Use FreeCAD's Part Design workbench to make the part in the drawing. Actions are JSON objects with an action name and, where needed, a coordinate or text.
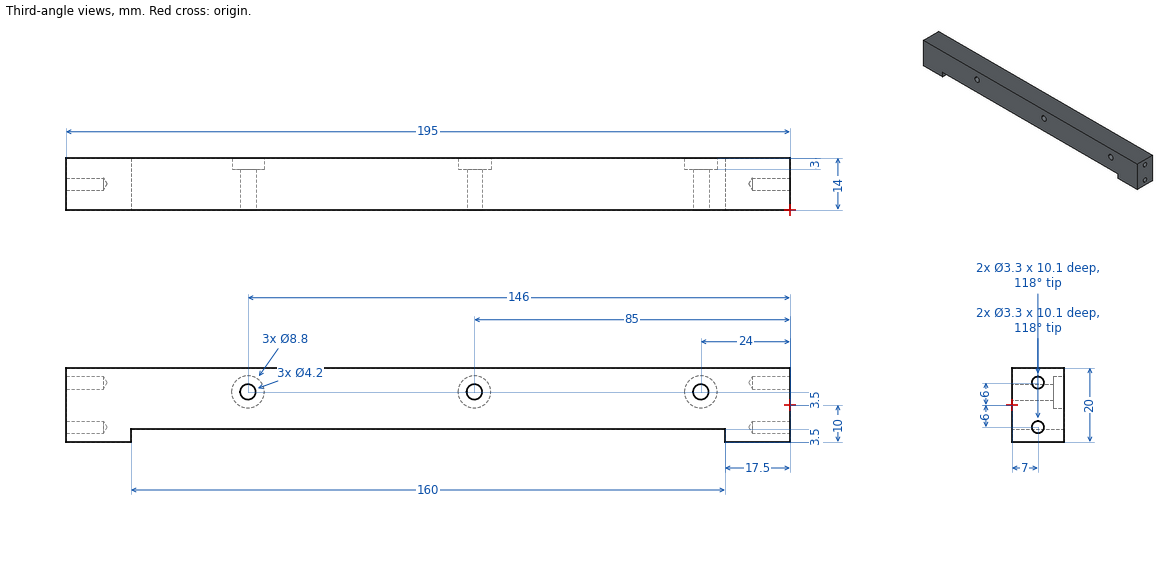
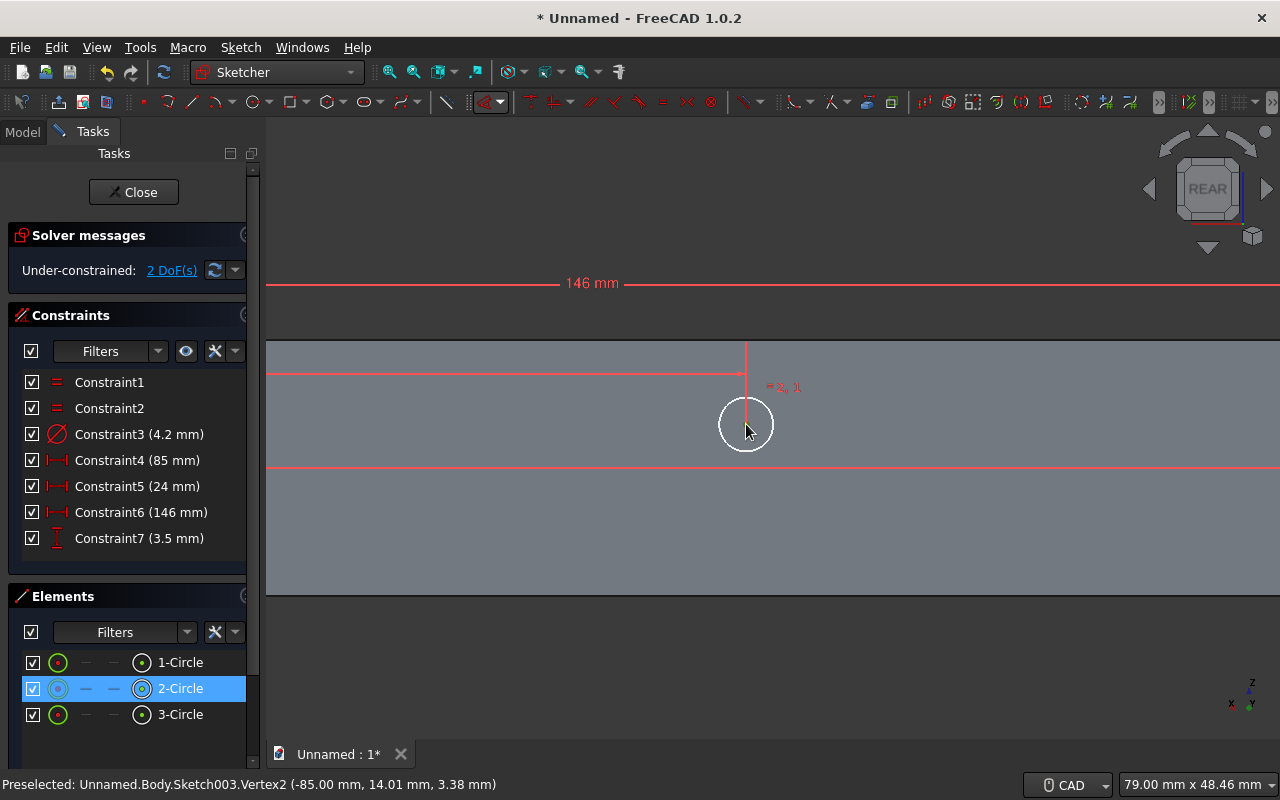
{"action": "left_click", "coordinate": [502, 102]}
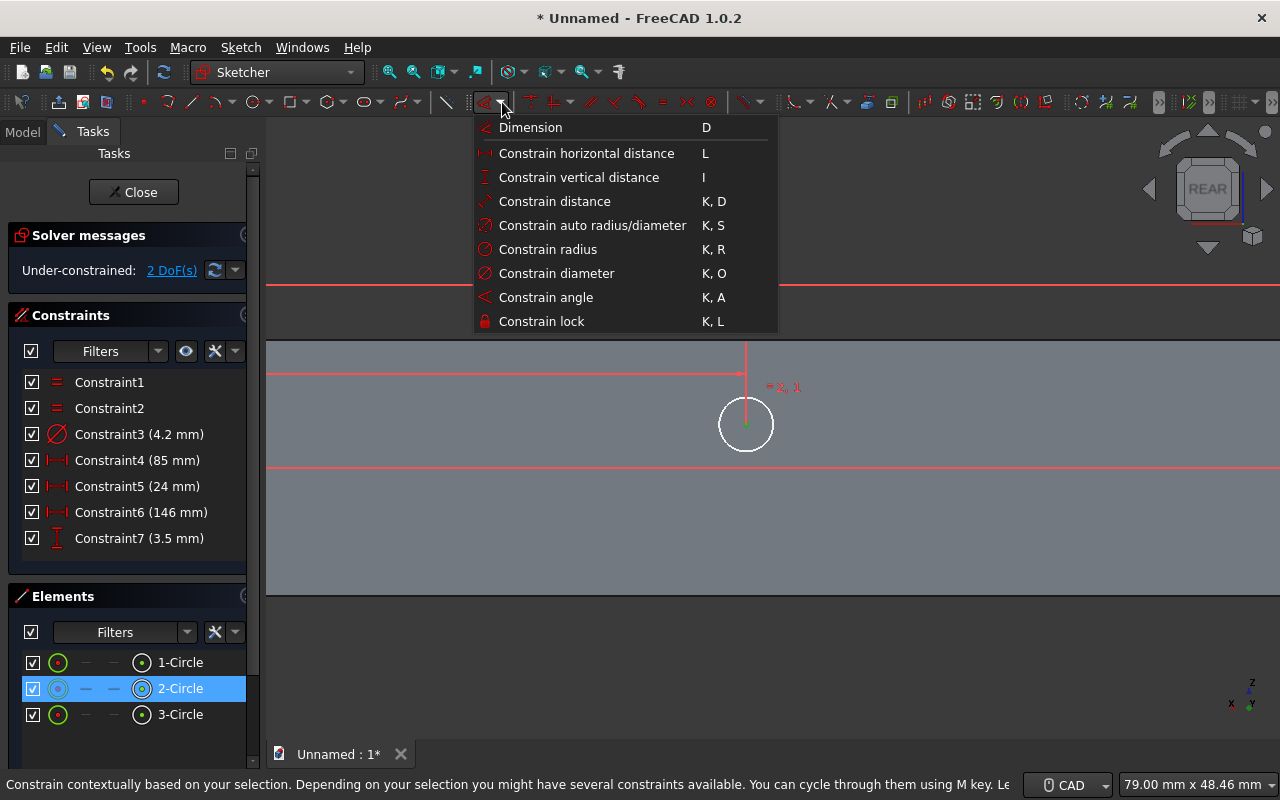
{"action": "left_click", "coordinate": [626, 177]}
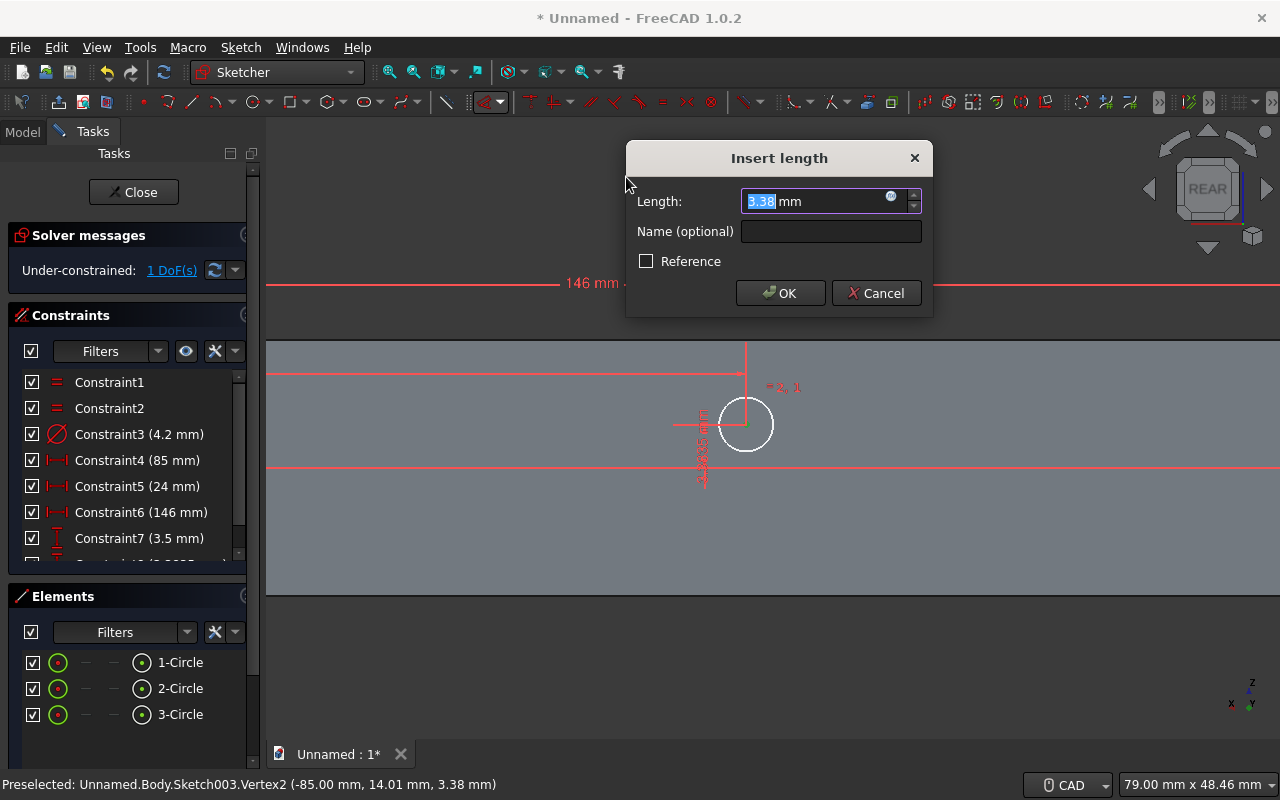
{"action": "type", "text": "3.5"}
{"action": "key", "text": "Return"}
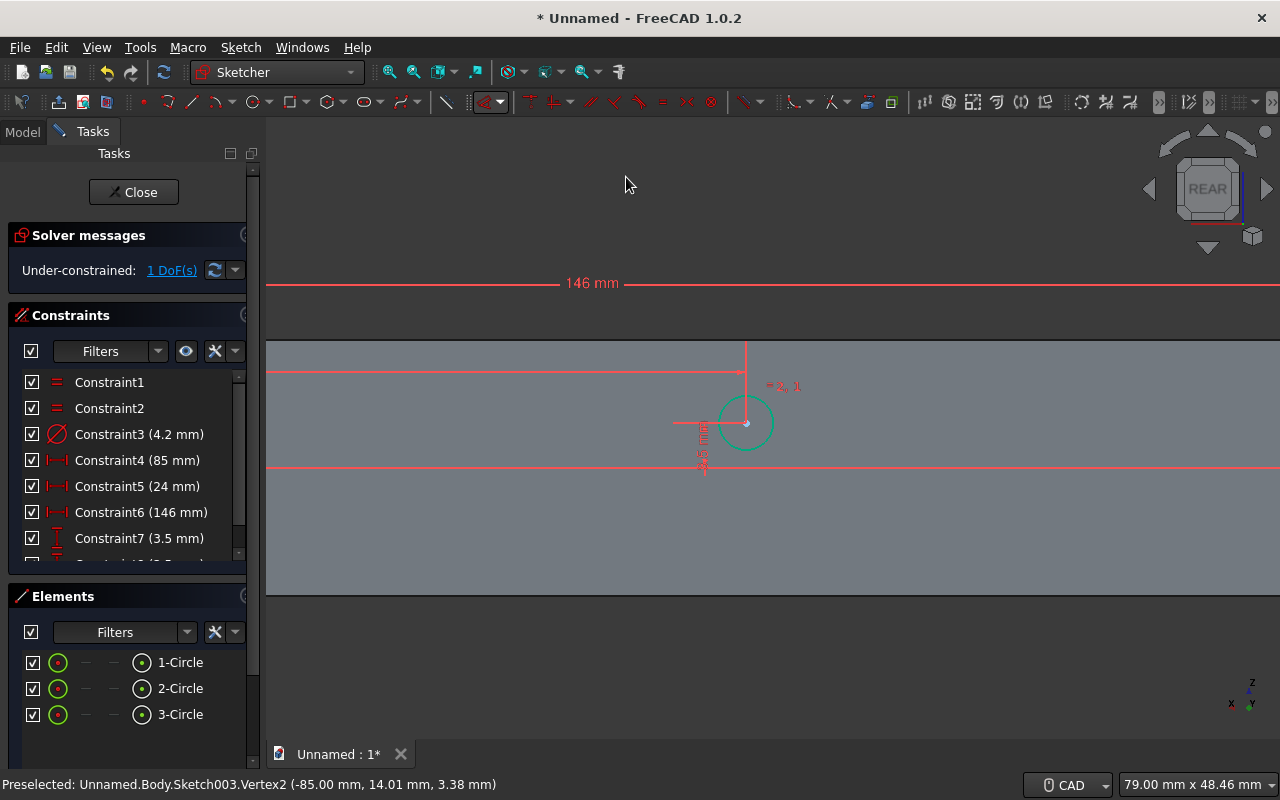
{"action": "scroll", "coordinate": [747, 426], "scroll_direction": "down", "scroll_amount": 6}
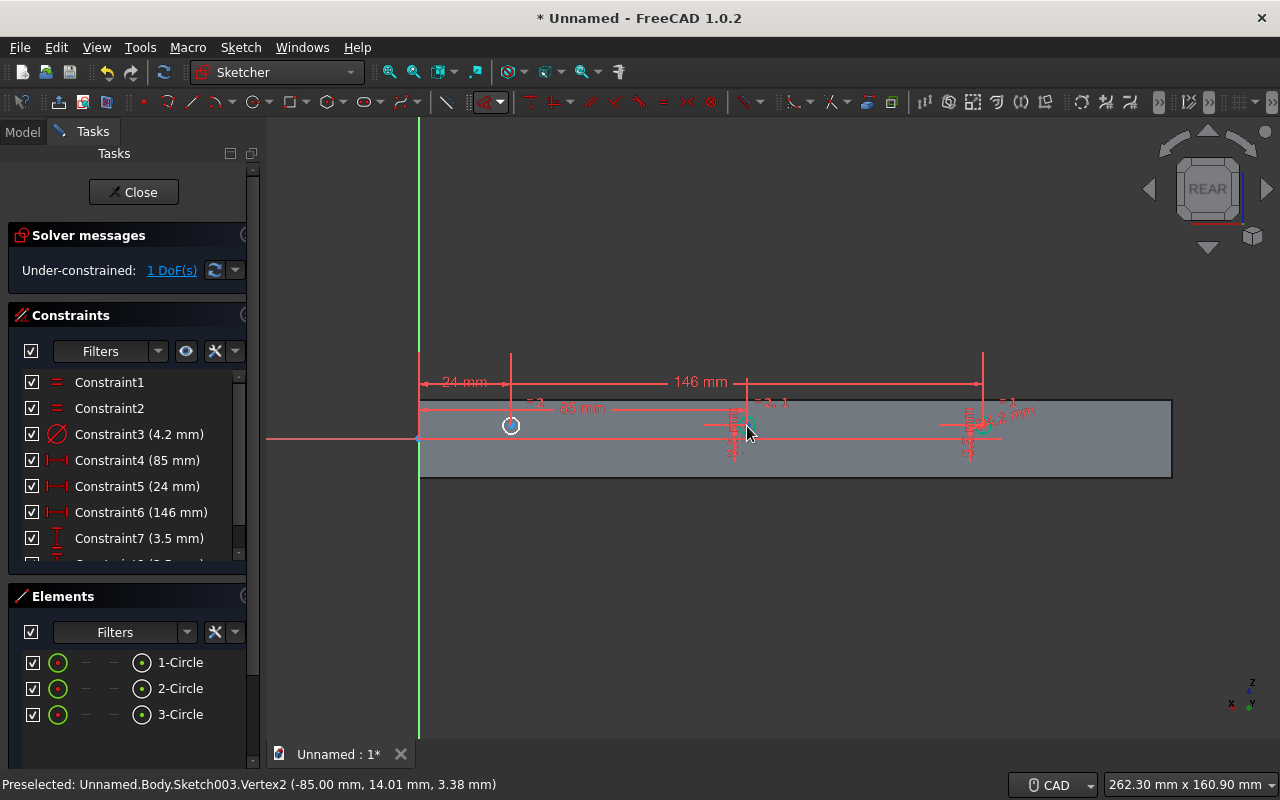
{"action": "scroll", "coordinate": [511, 426], "scroll_direction": "up", "scroll_amount": 6}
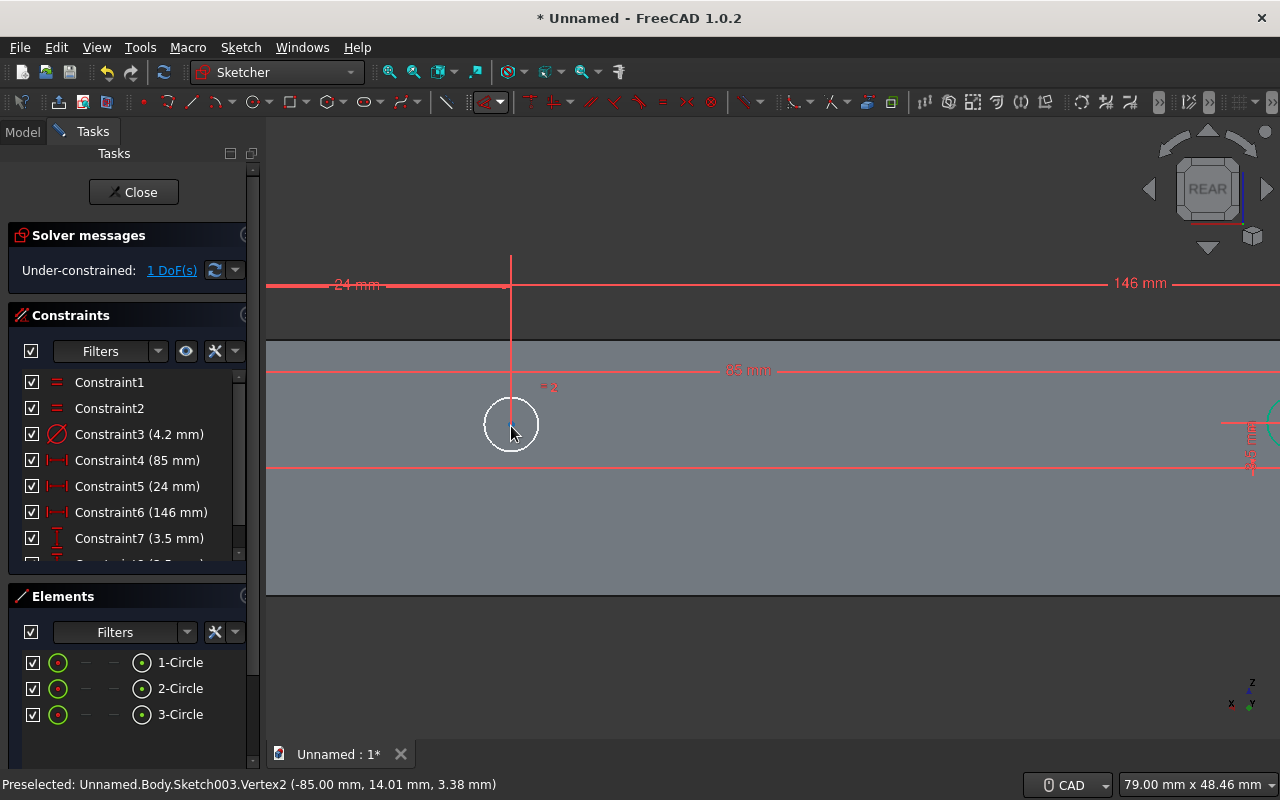
{"action": "left_click", "coordinate": [511, 424]}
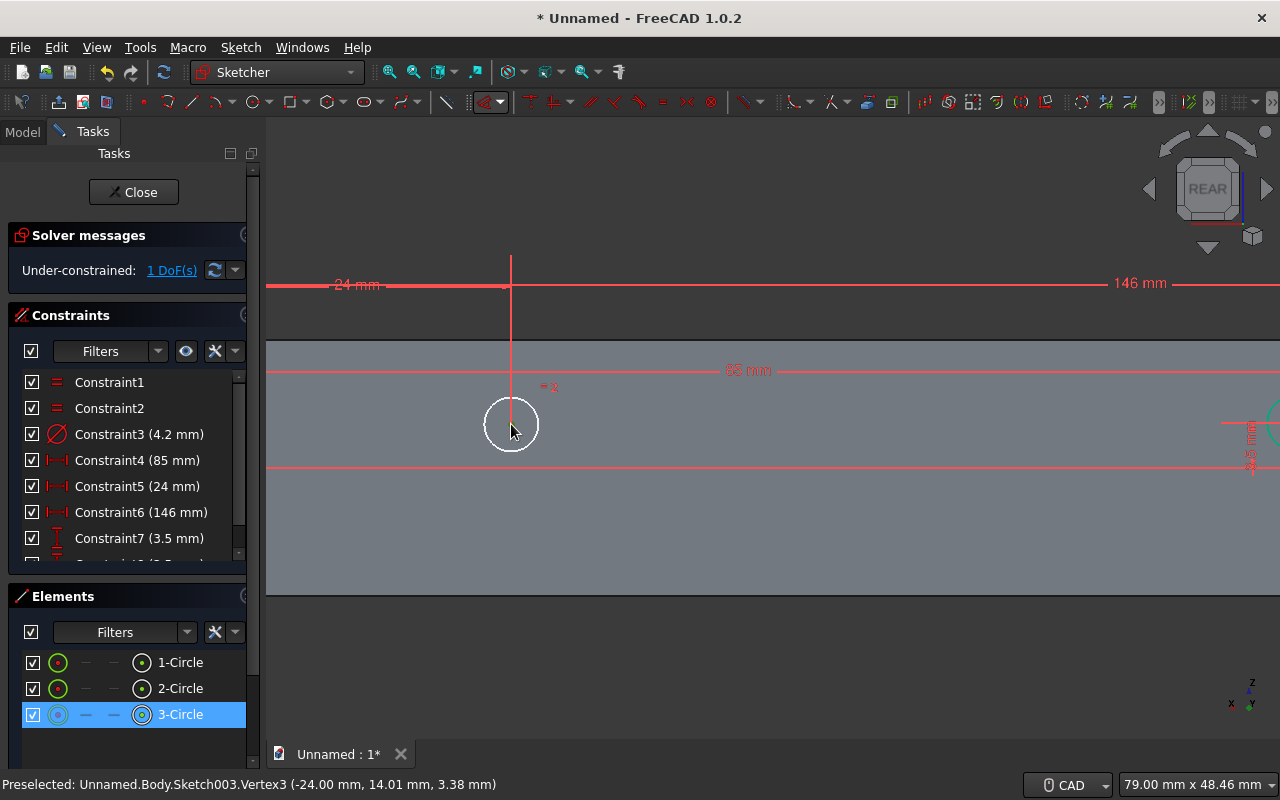
{"action": "key", "text": "i"}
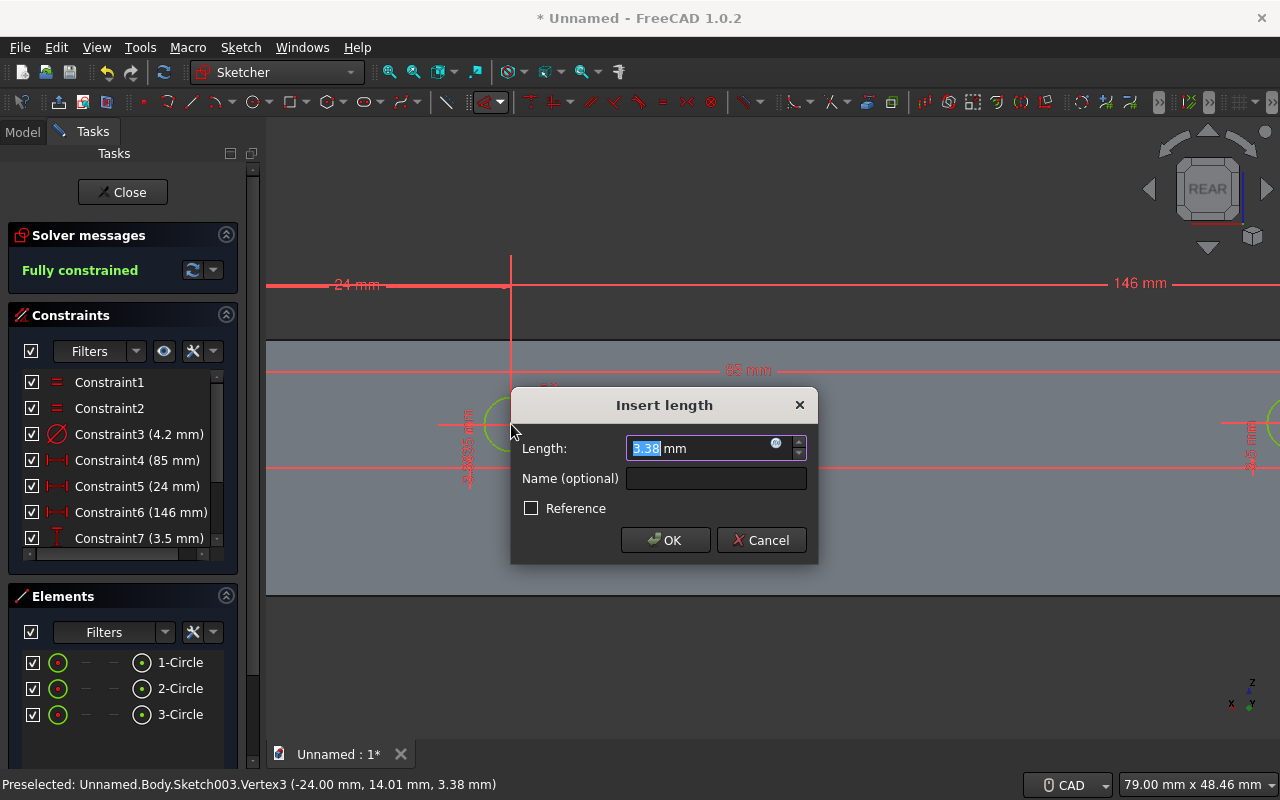
{"action": "type", "text": "3.5"}
{"action": "key", "text": "Return"}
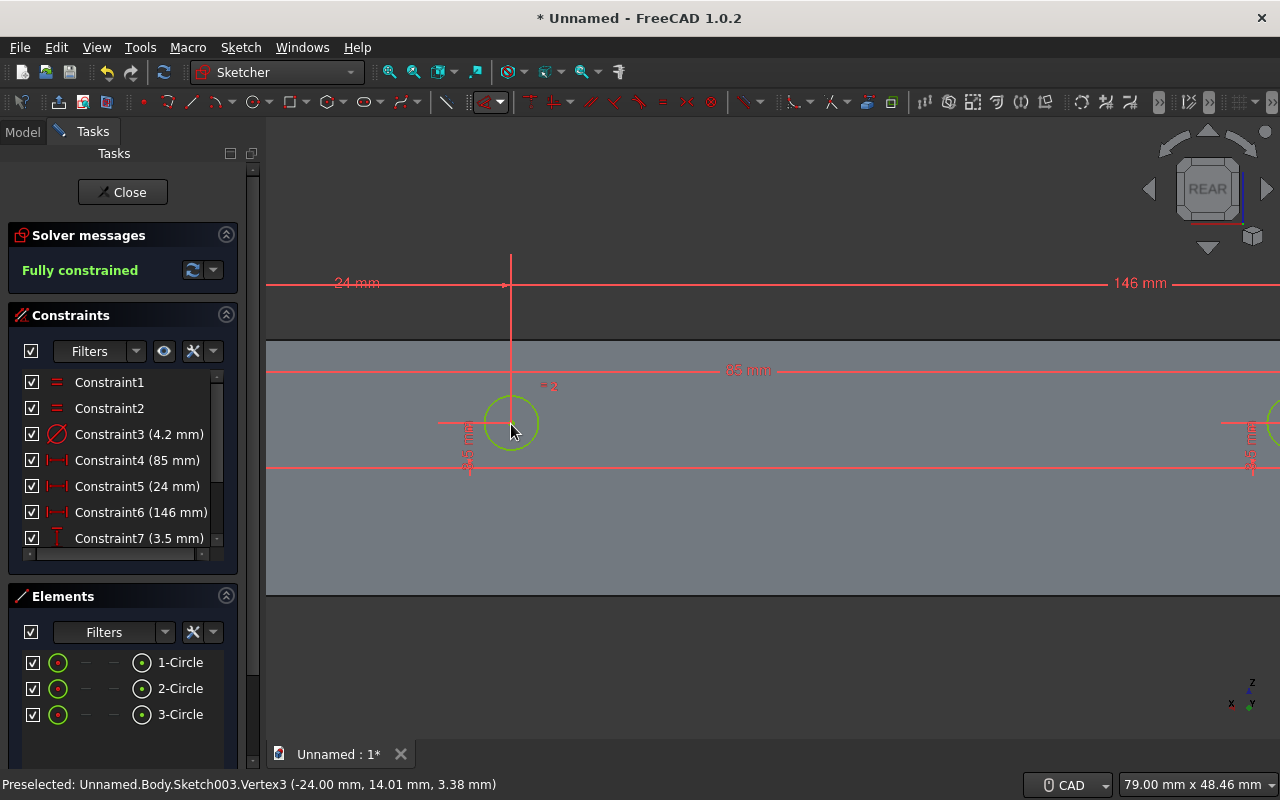
{"action": "left_click", "coordinate": [123, 192]}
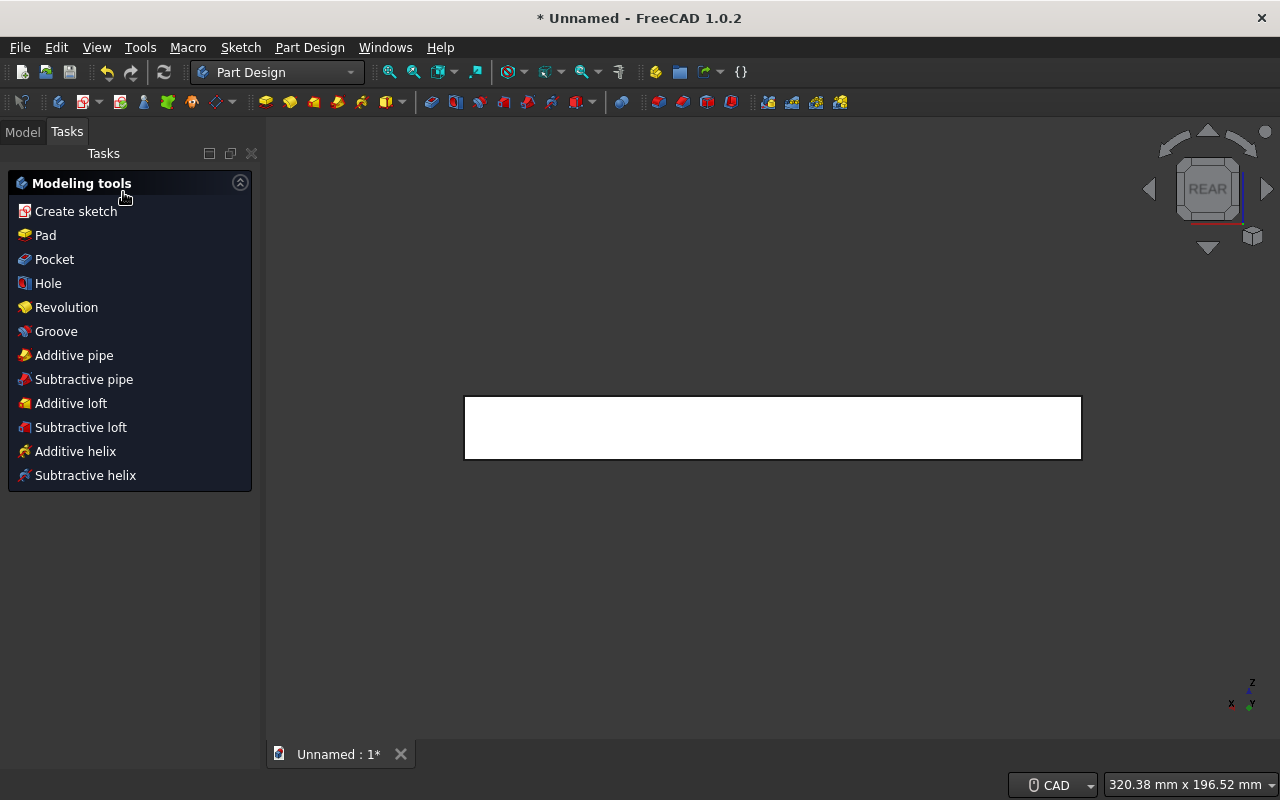
{"action": "left_click", "coordinate": [432, 102]}